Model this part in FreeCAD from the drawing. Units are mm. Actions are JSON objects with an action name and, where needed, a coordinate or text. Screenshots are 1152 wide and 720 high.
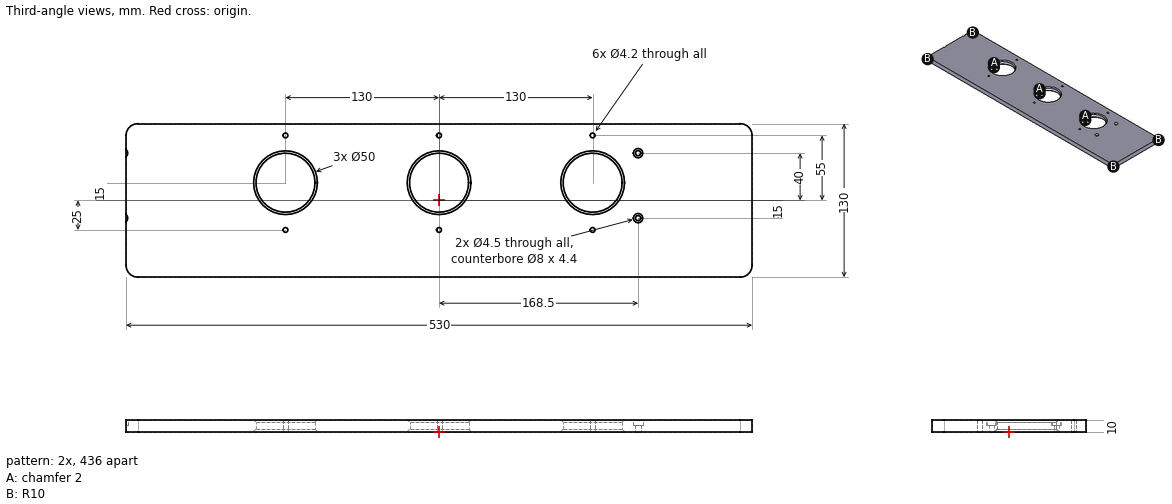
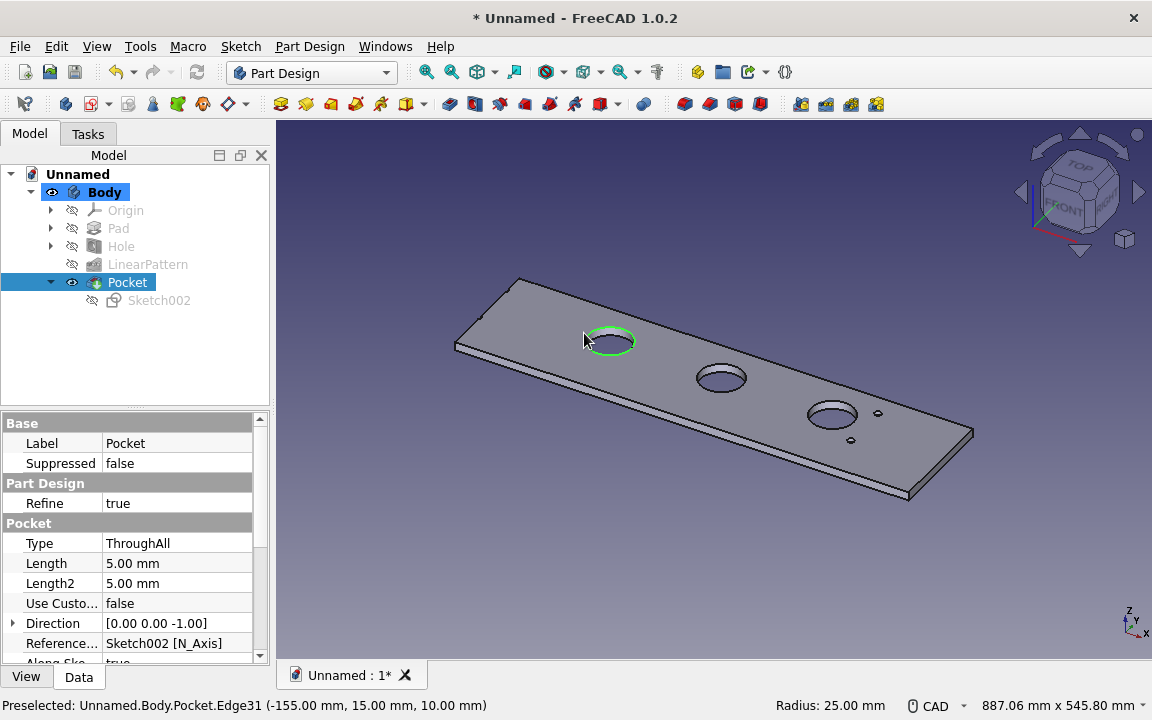
{"action": "left_click", "coordinate": [700, 370], "text": "ctrl"}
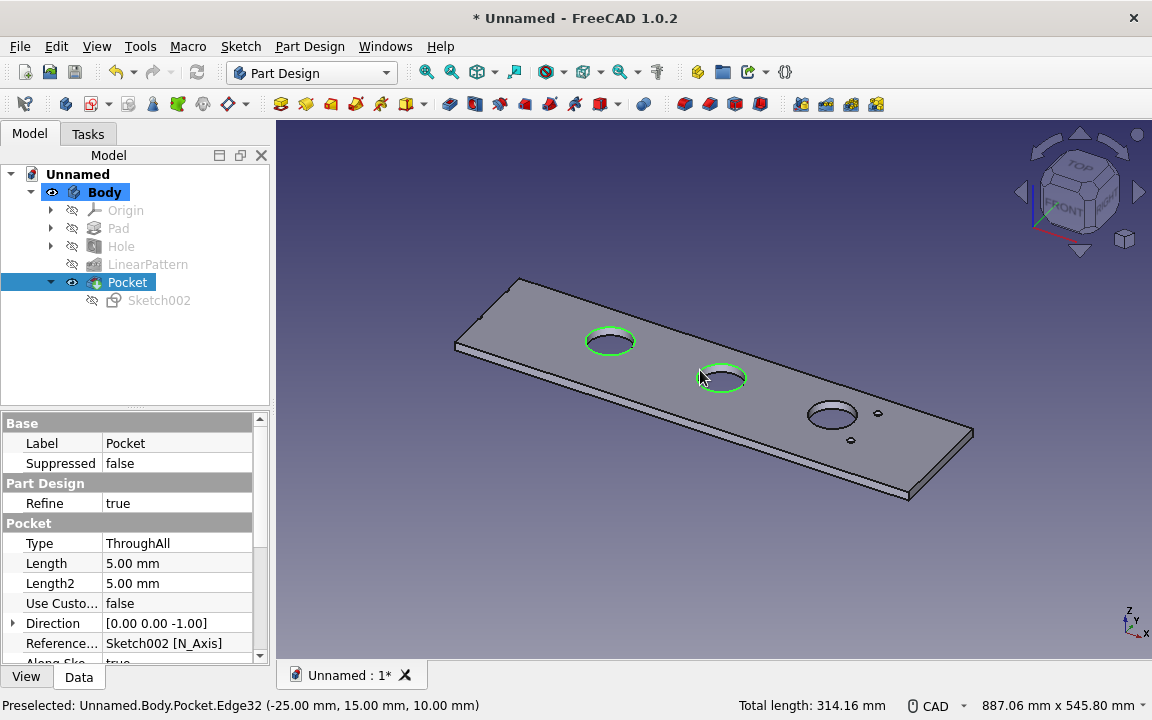
{"action": "left_click", "coordinate": [811, 407], "text": "ctrl"}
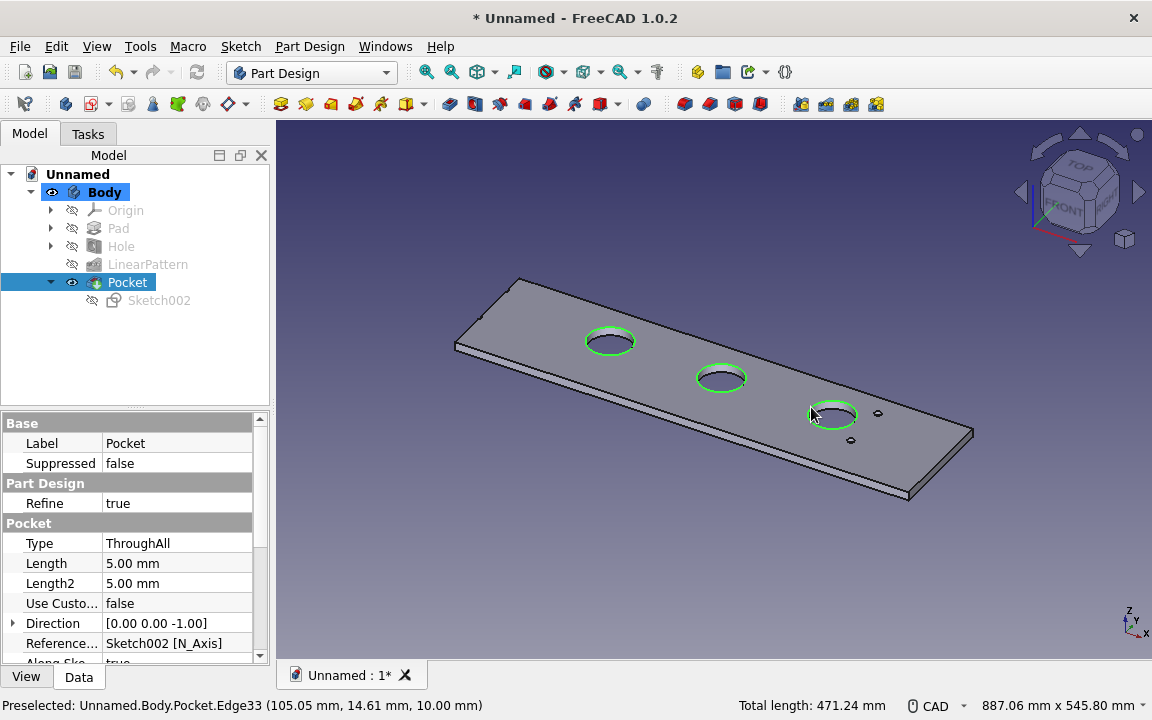
{"action": "key", "text": "0"}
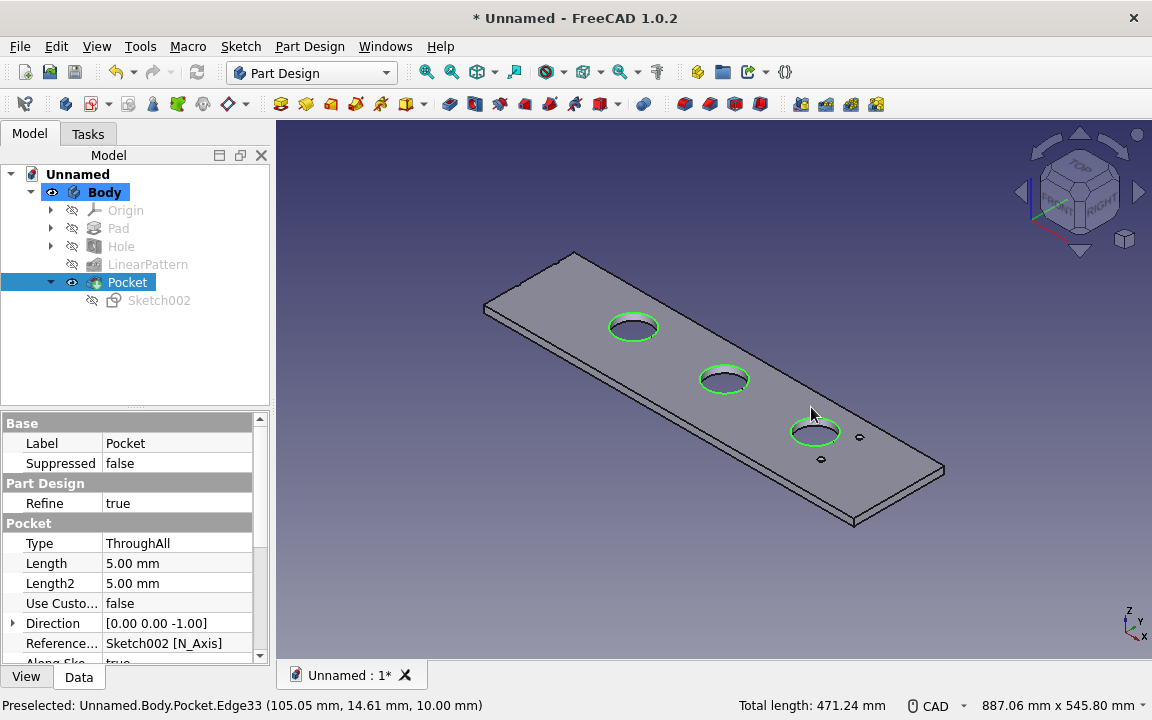
{"action": "key", "text": "2"}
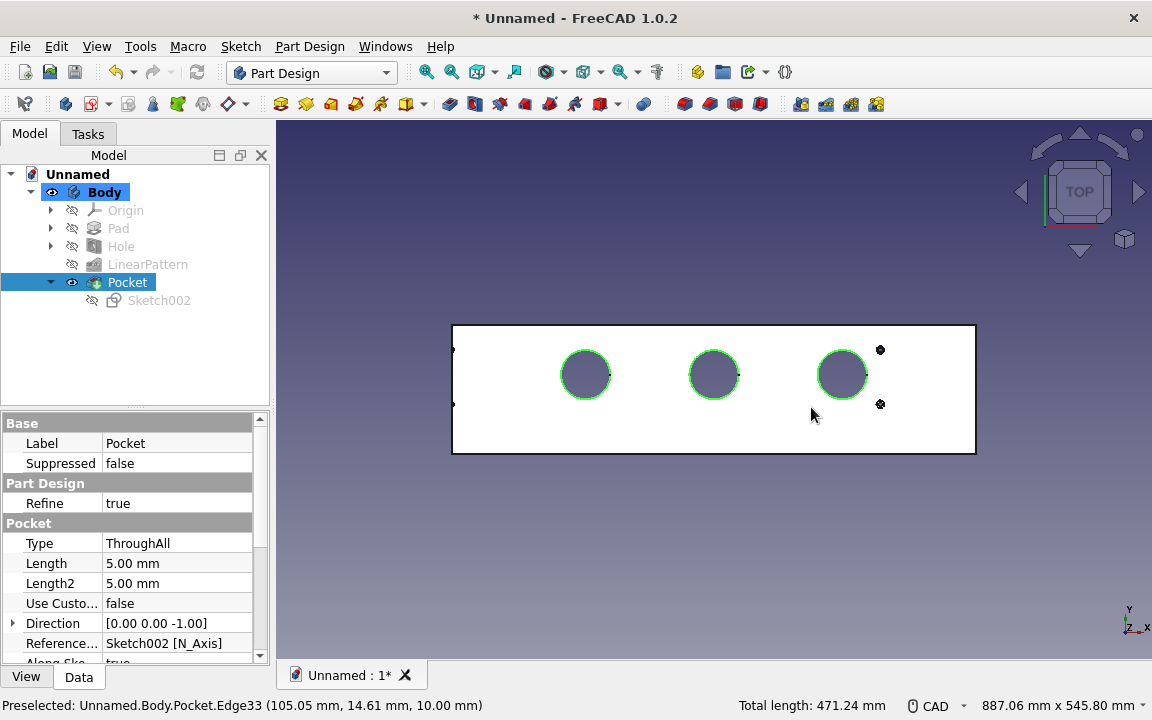
{"action": "key", "text": "1"}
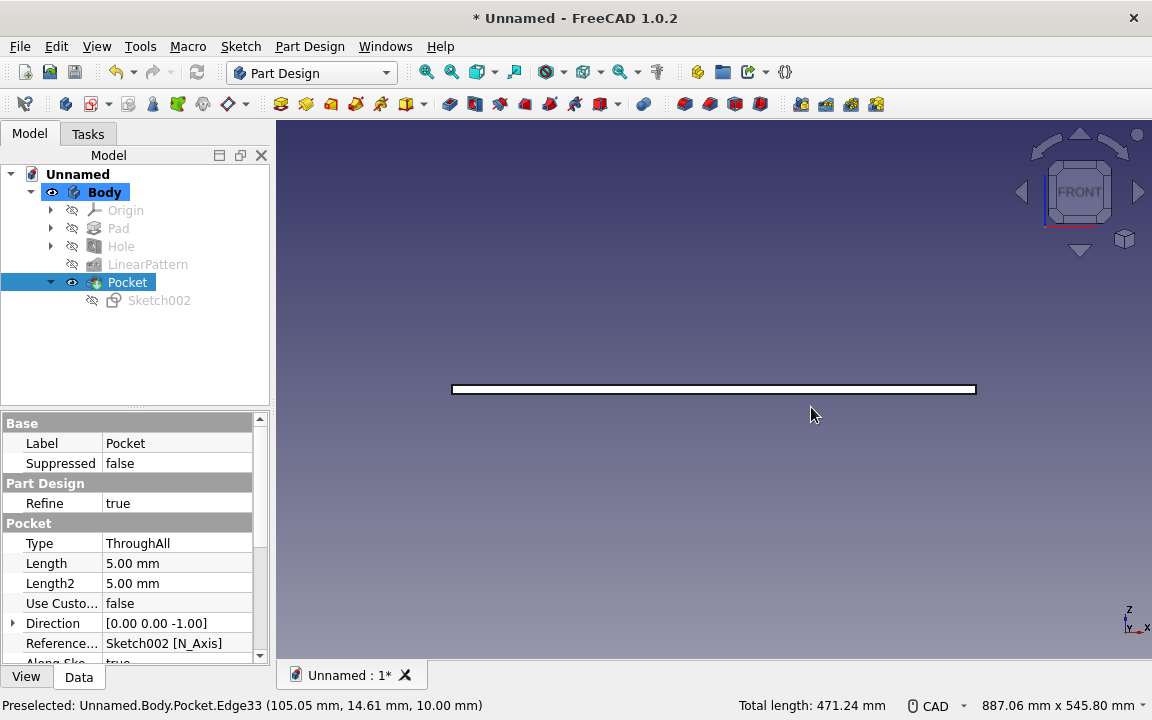
{"action": "key", "text": "3"}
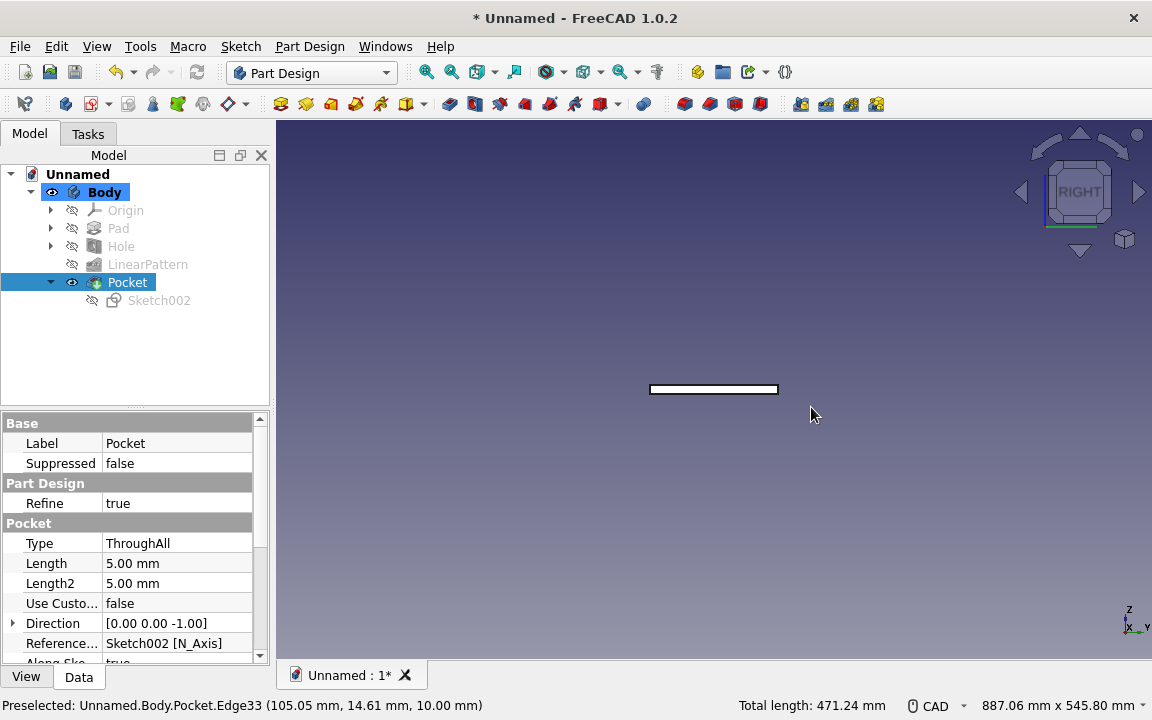
{"action": "left_click", "coordinate": [427, 72]}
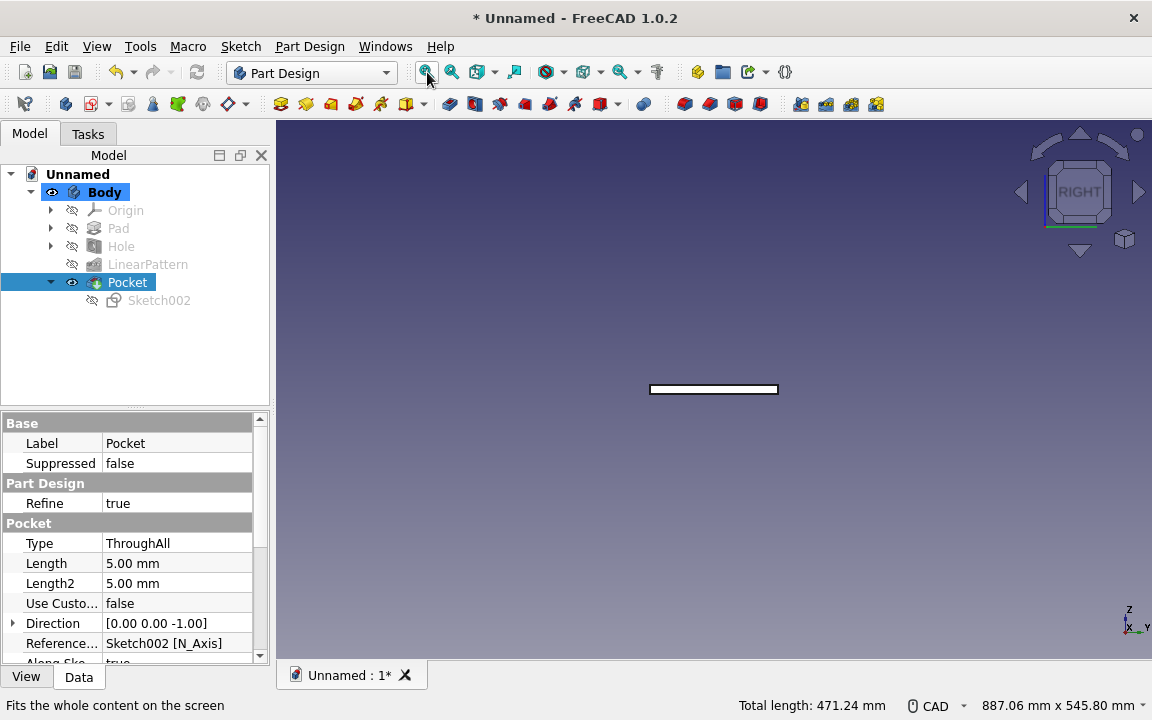
{"action": "key", "text": "5"}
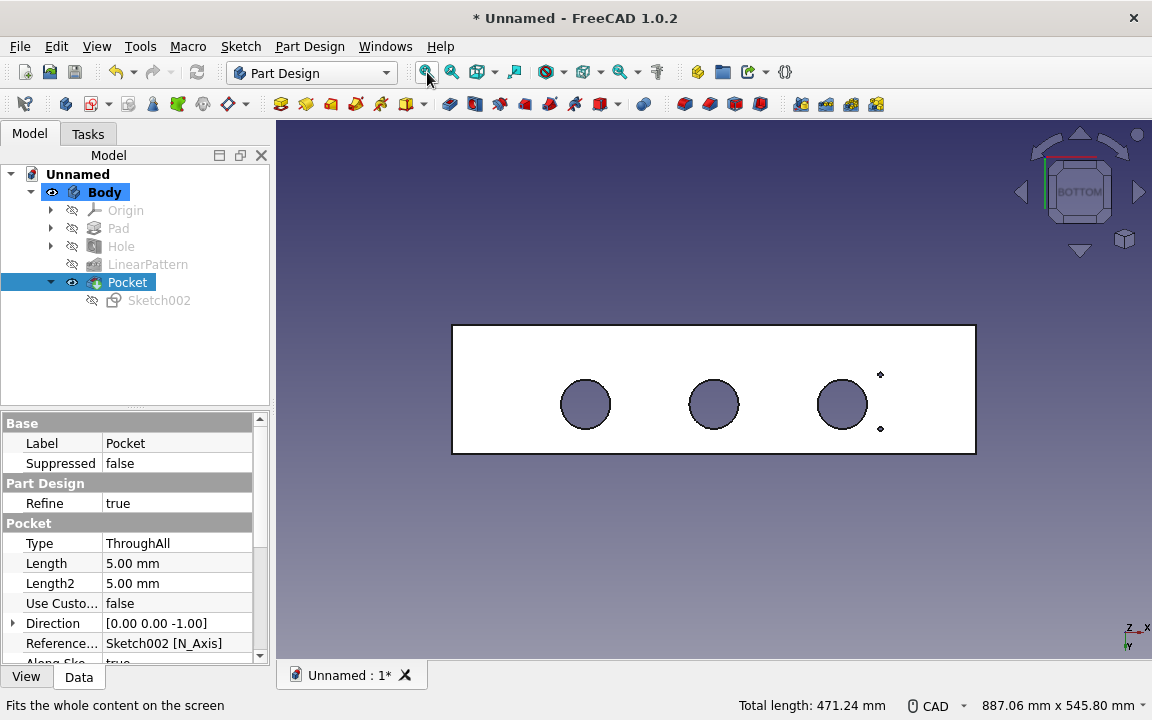
{"action": "left_click", "coordinate": [561, 403], "text": "ctrl"}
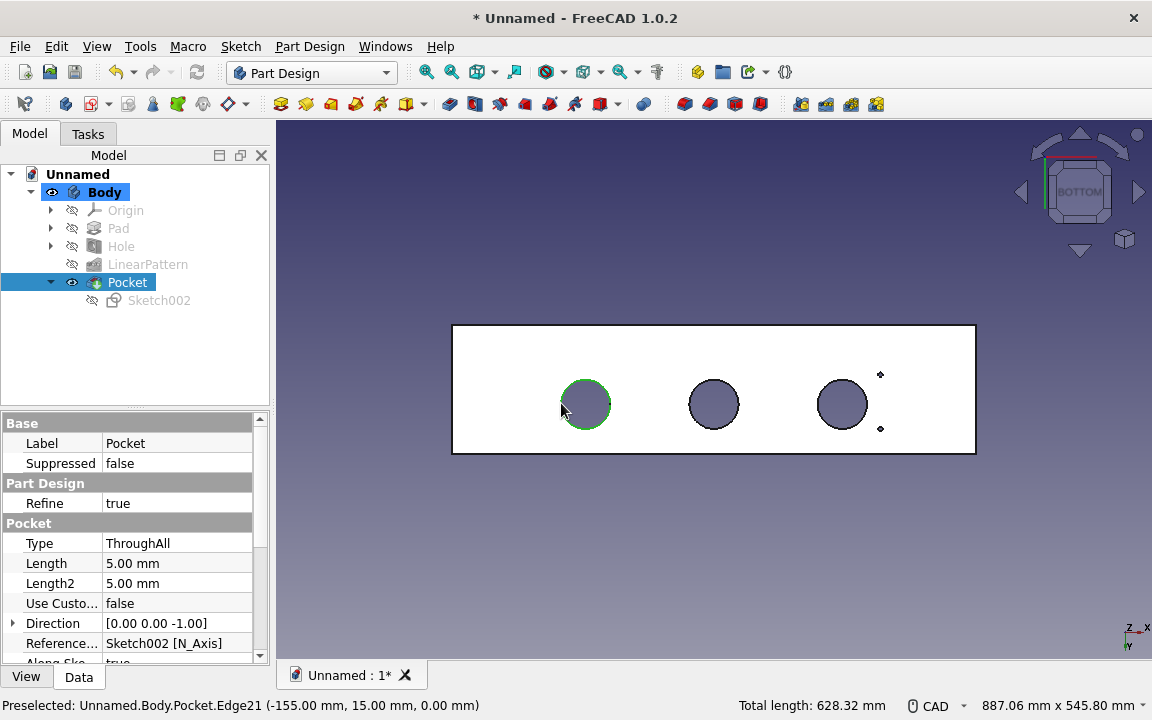
{"action": "left_click", "coordinate": [694, 418], "text": "ctrl"}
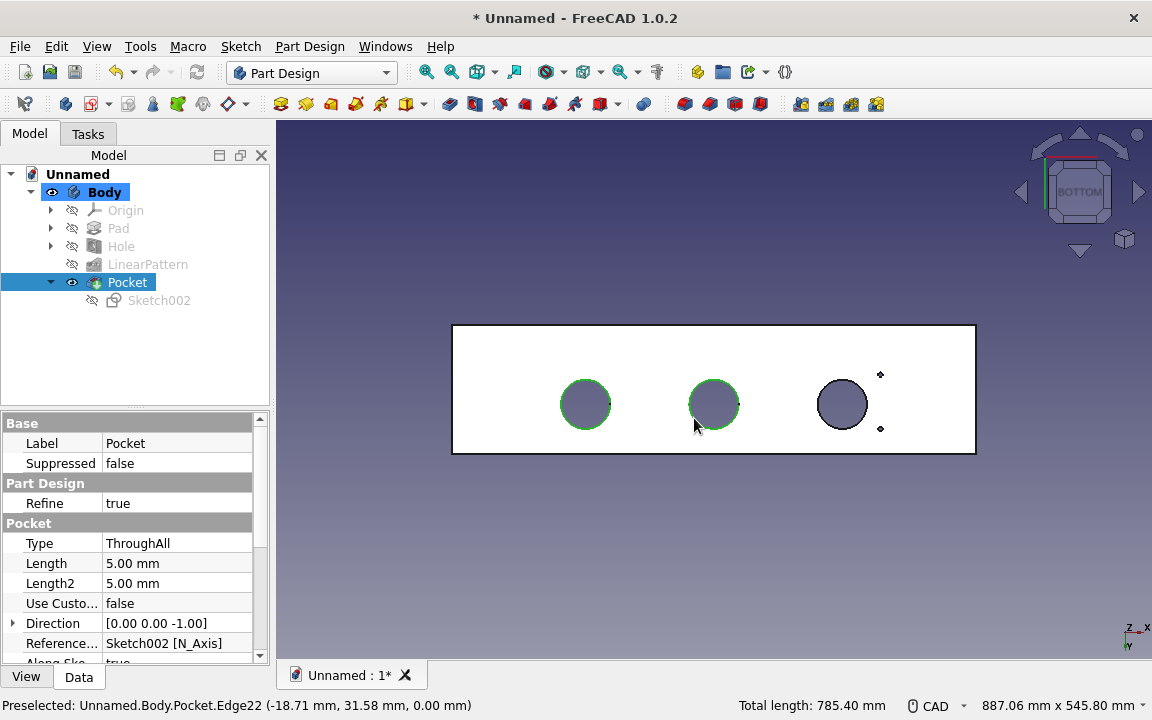
{"action": "left_click", "coordinate": [822, 418], "text": "ctrl"}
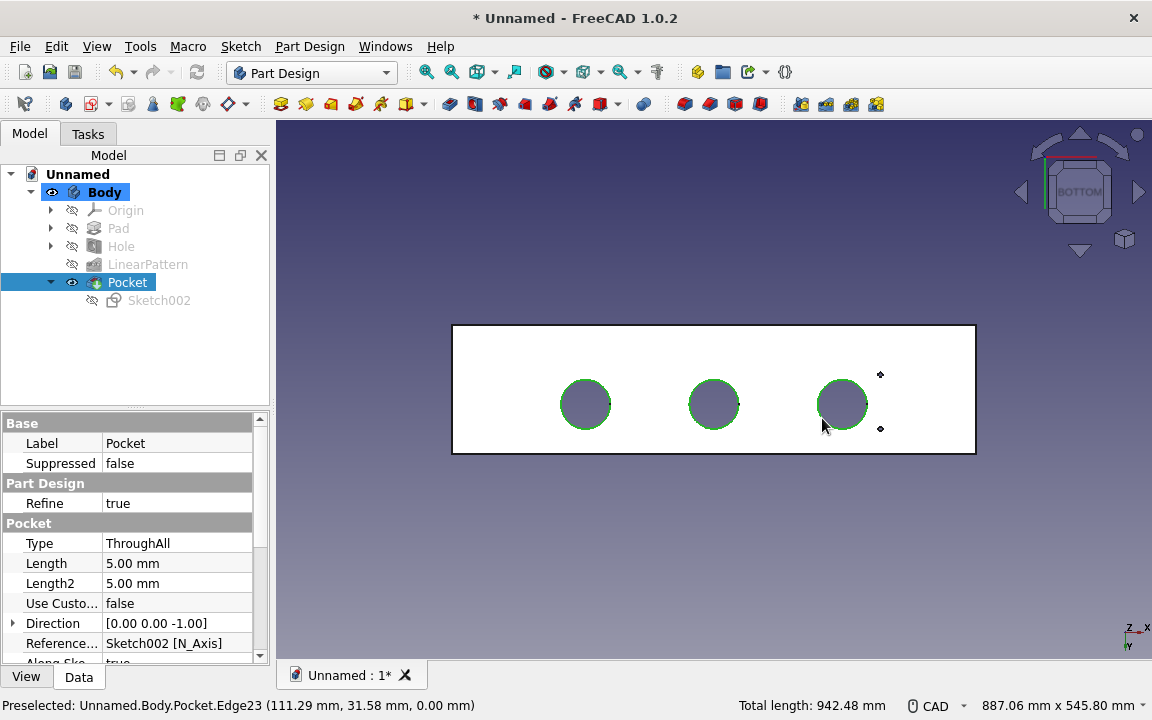
{"action": "left_click", "coordinate": [710, 104]}